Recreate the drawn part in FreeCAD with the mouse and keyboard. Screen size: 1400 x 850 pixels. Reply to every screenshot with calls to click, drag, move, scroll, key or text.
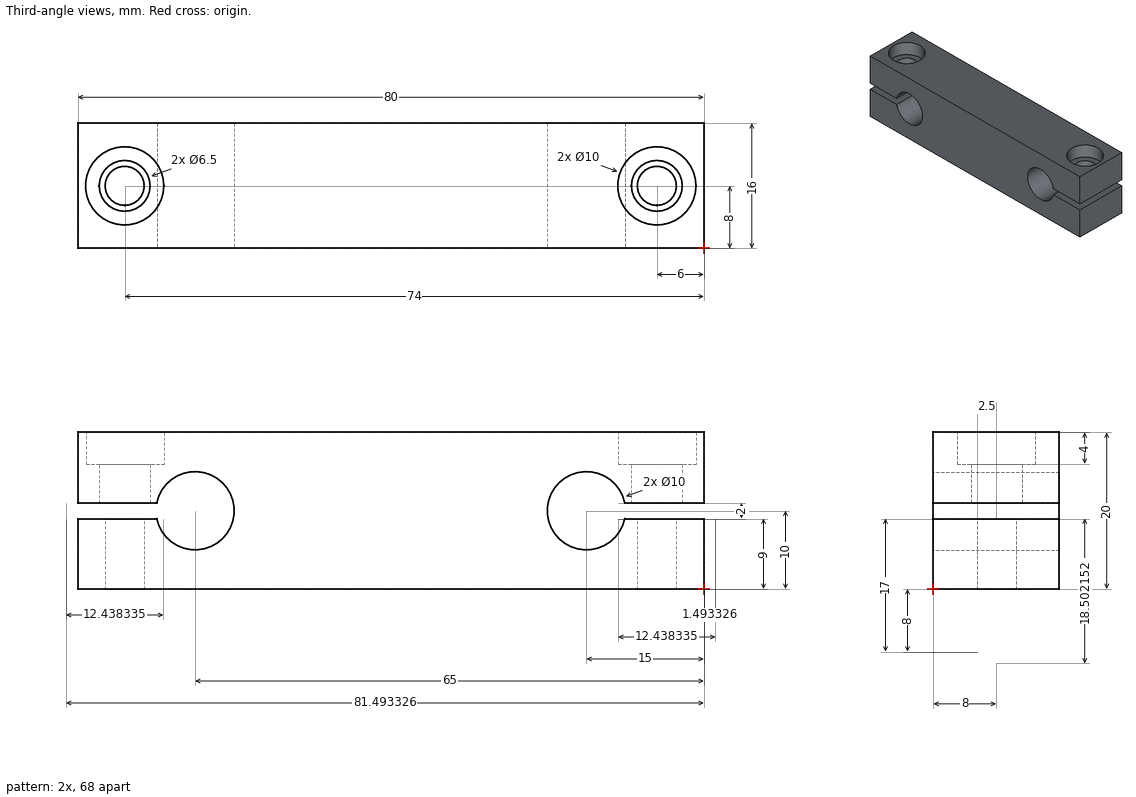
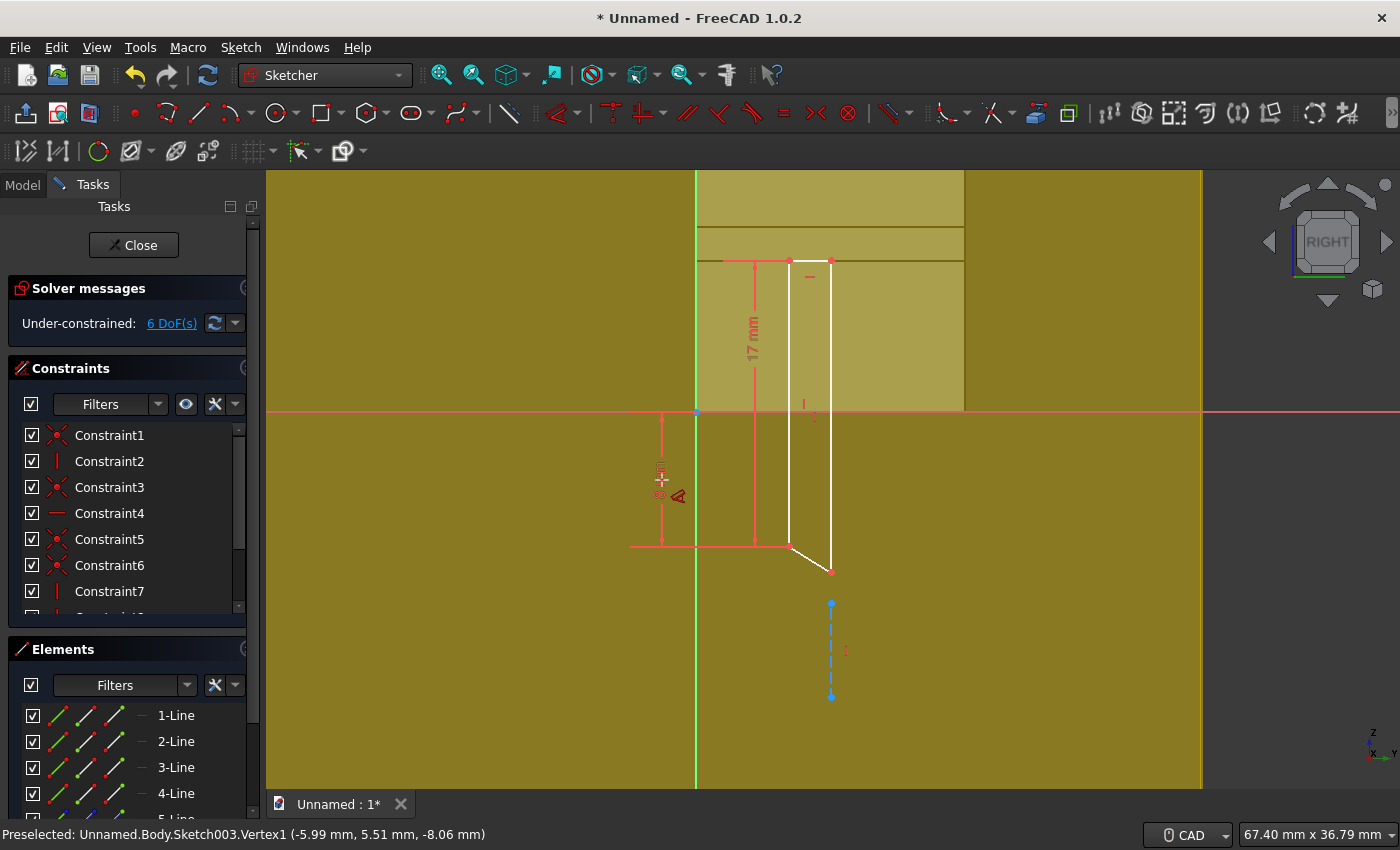
click(831, 573)
click(764, 607)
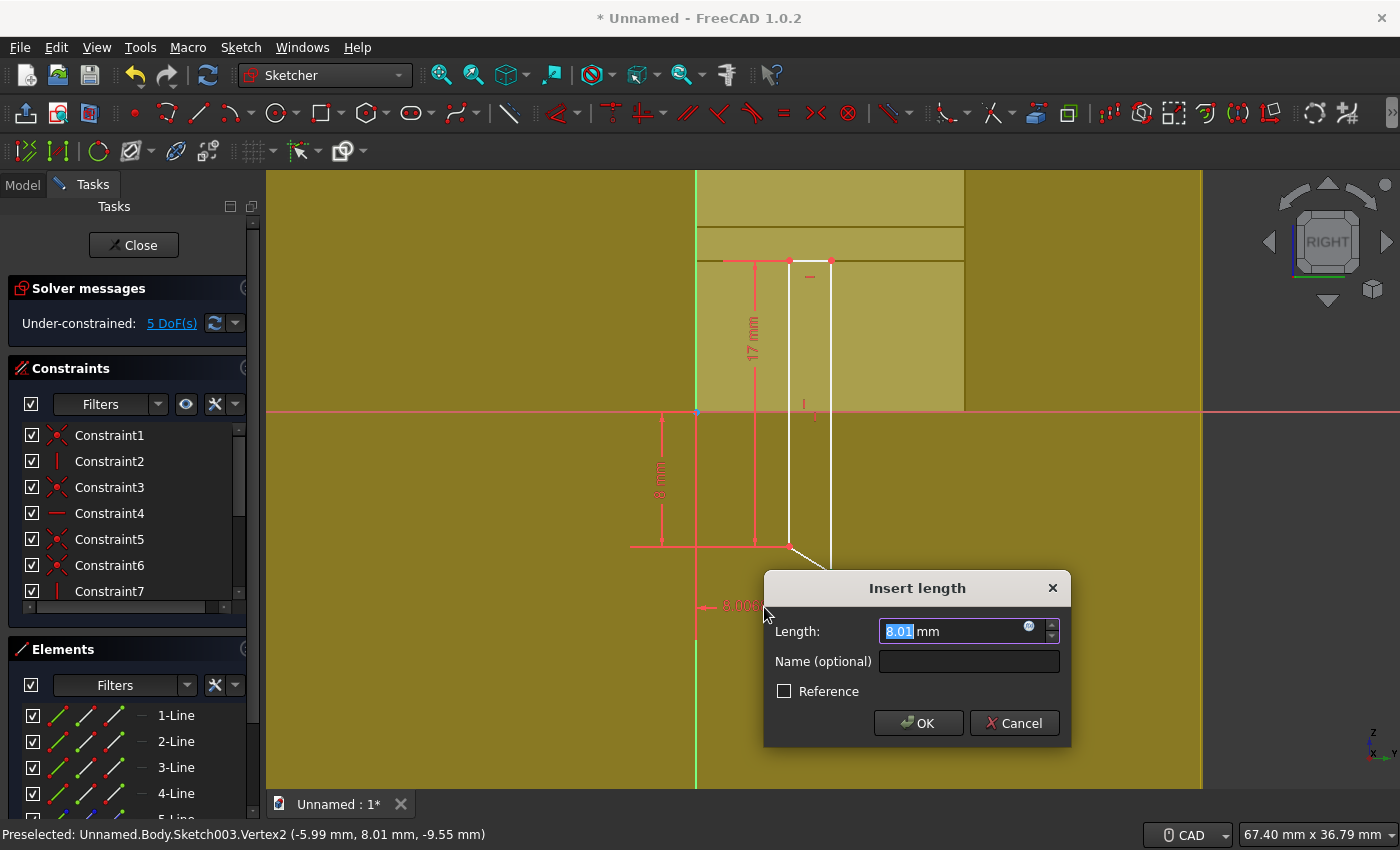
text(8)
key(Return)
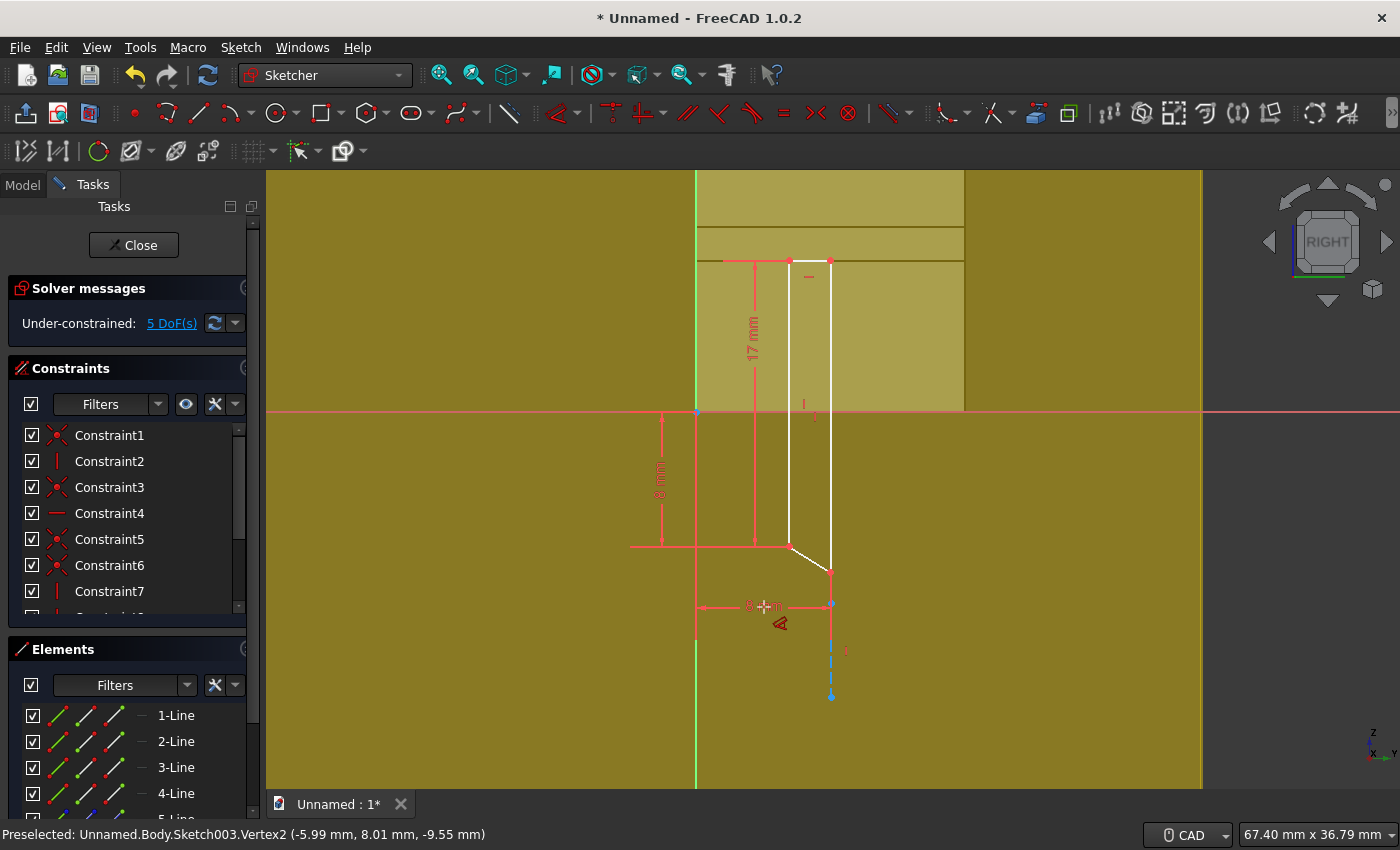
click(831, 604)
click(764, 638)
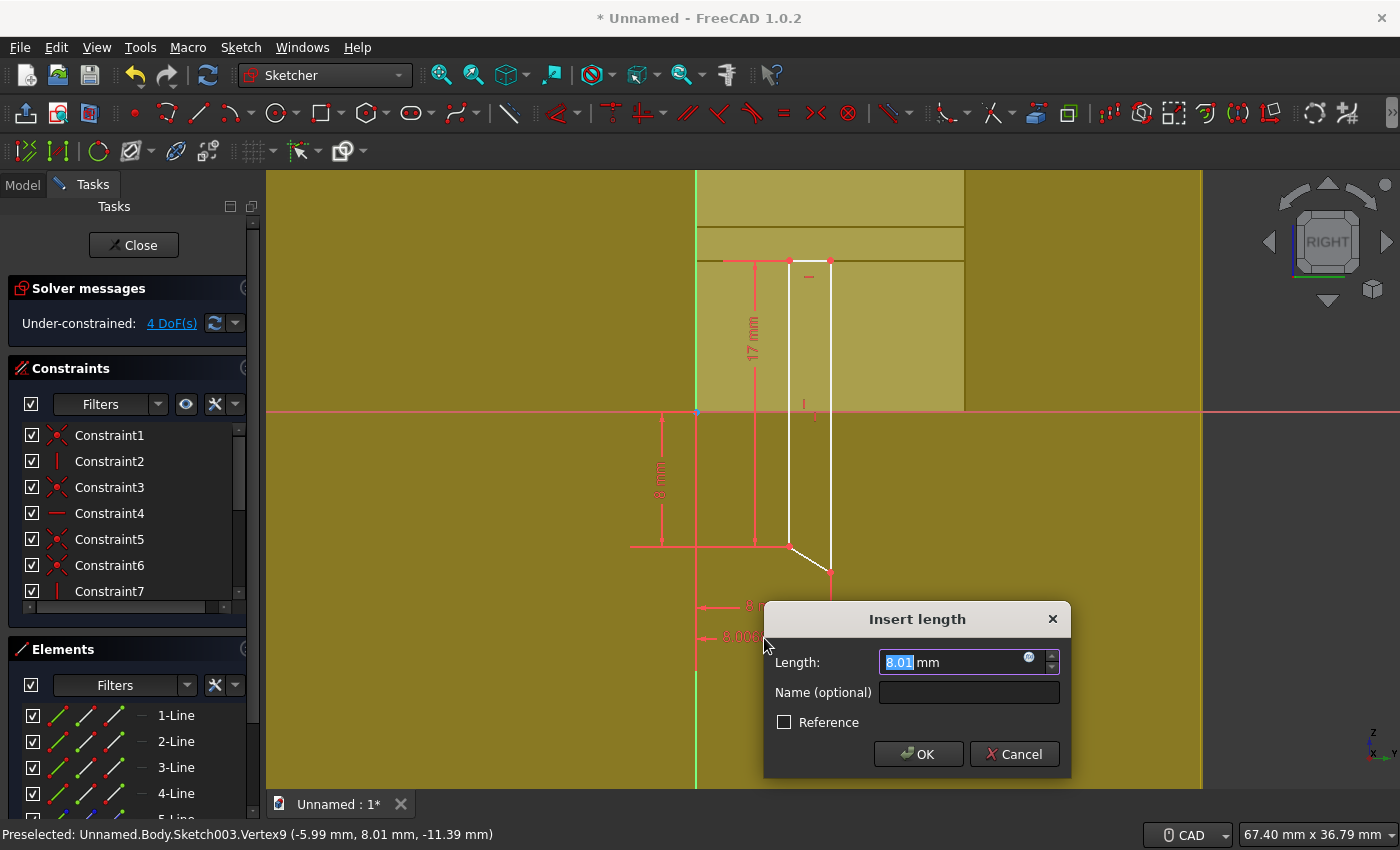
text(8)
key(Return)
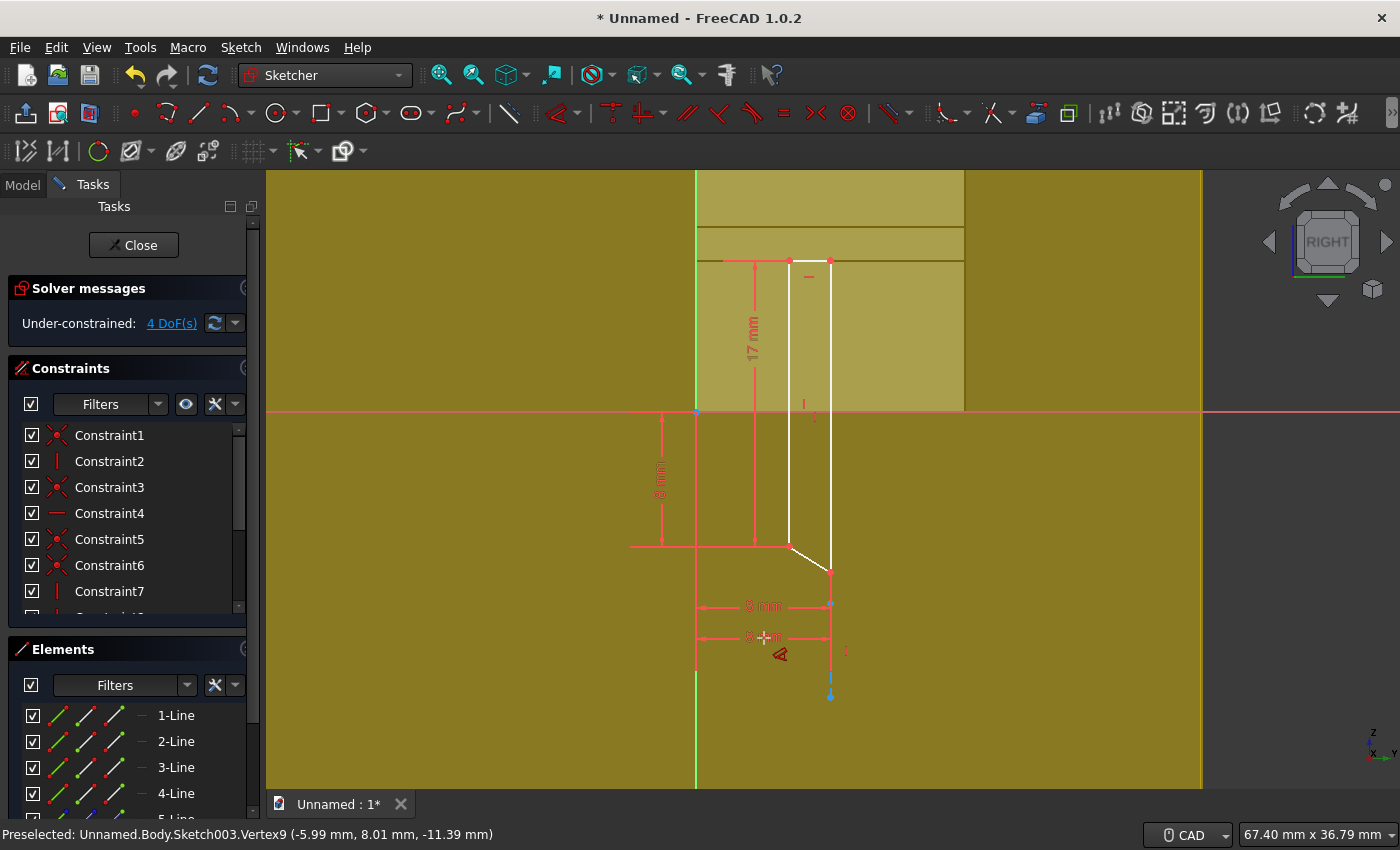
click(818, 261)
click(810, 227)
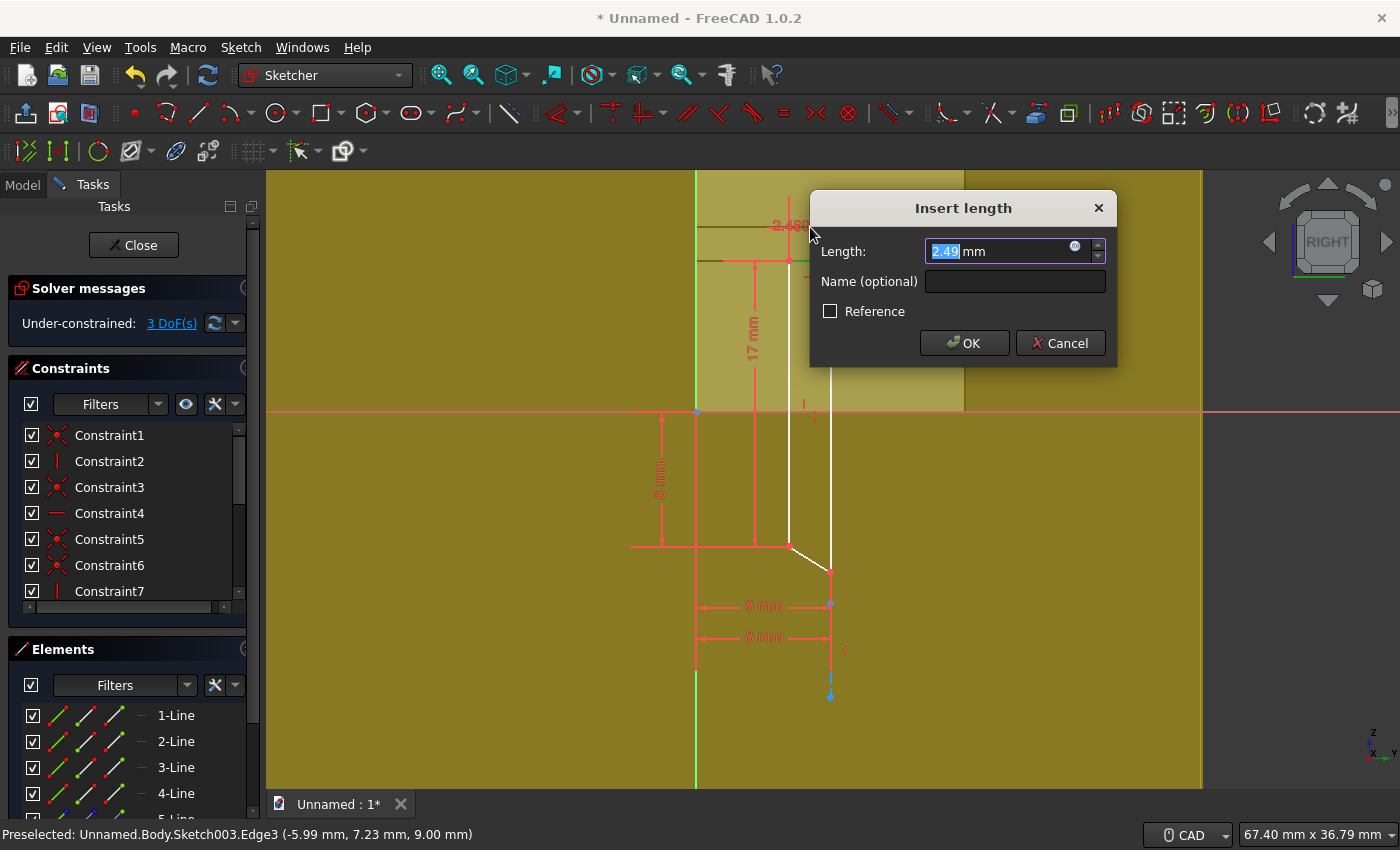
text(2.5)
key(Return)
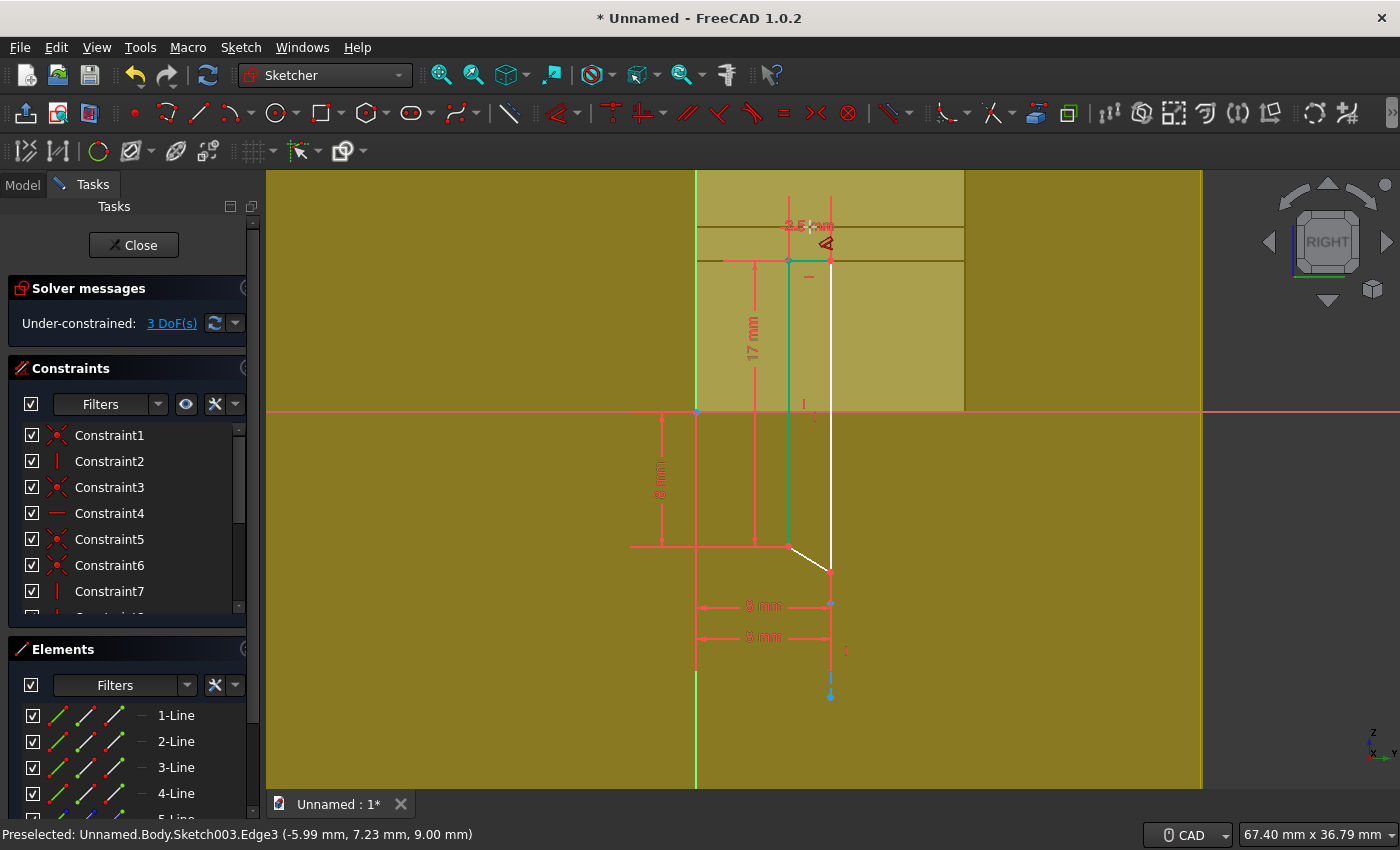
click(831, 479)
click(865, 345)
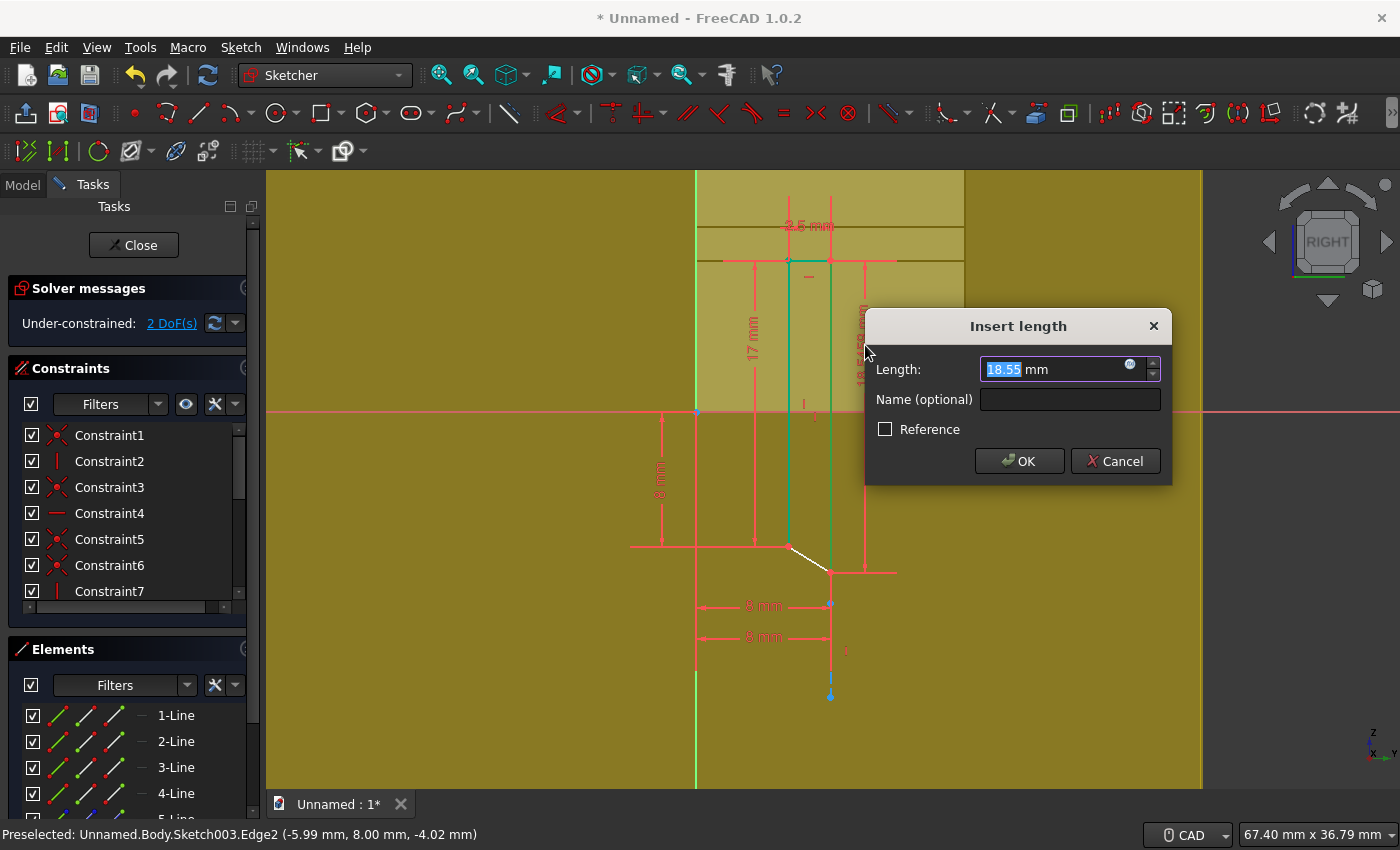
text(18.502152)
key(Return)
key(Escape)